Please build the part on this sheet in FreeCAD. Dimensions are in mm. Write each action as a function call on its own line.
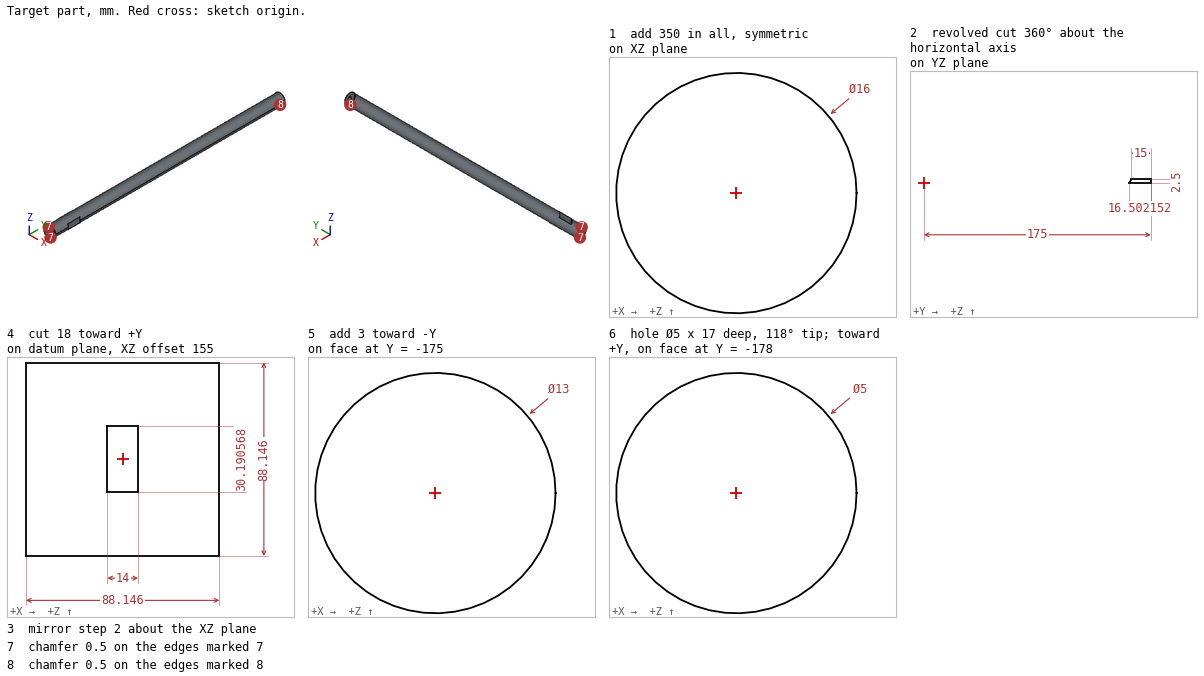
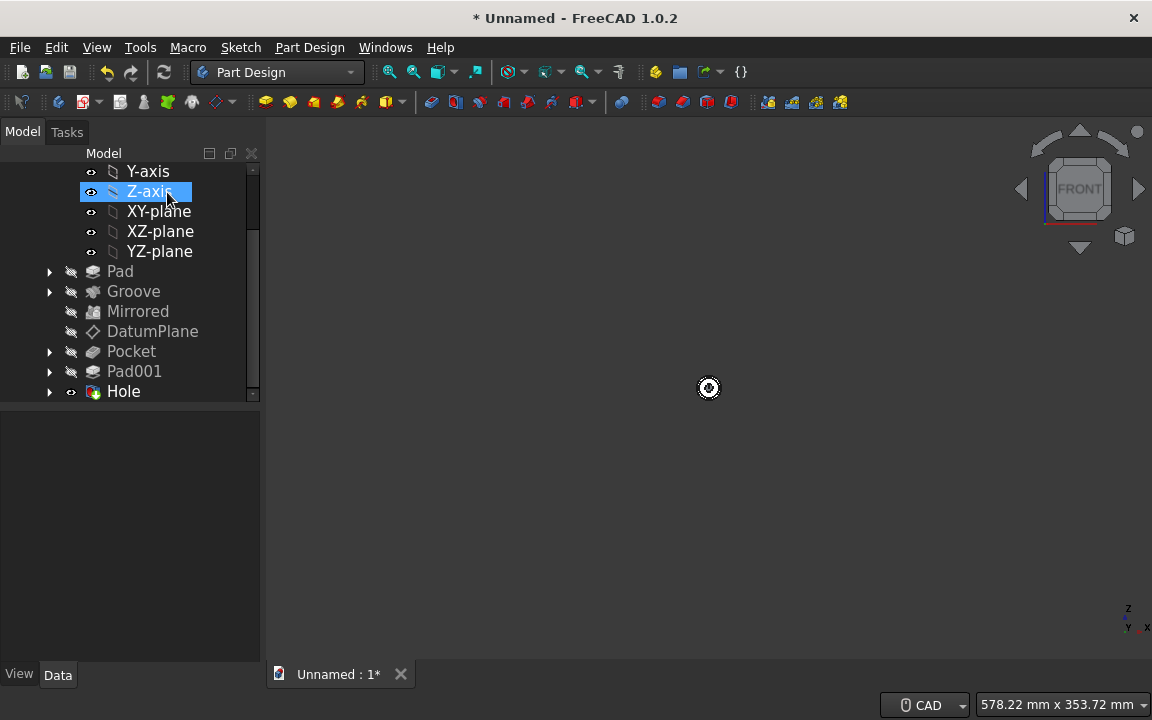
click(390, 72)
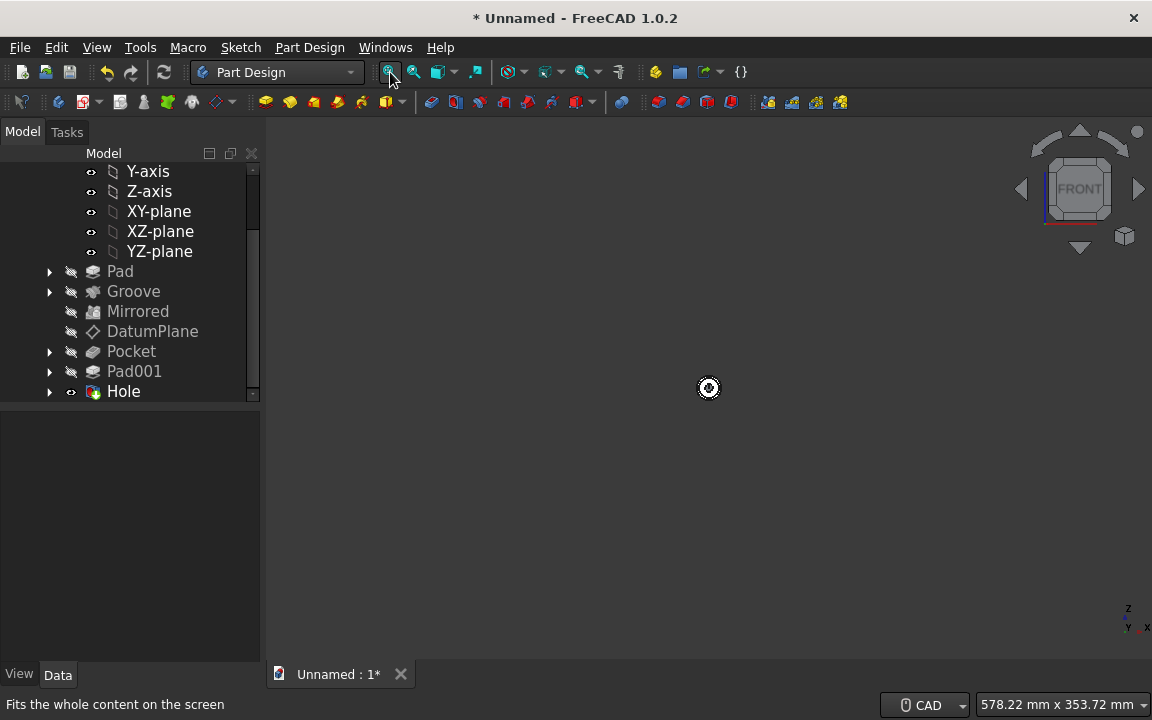
click(699, 387)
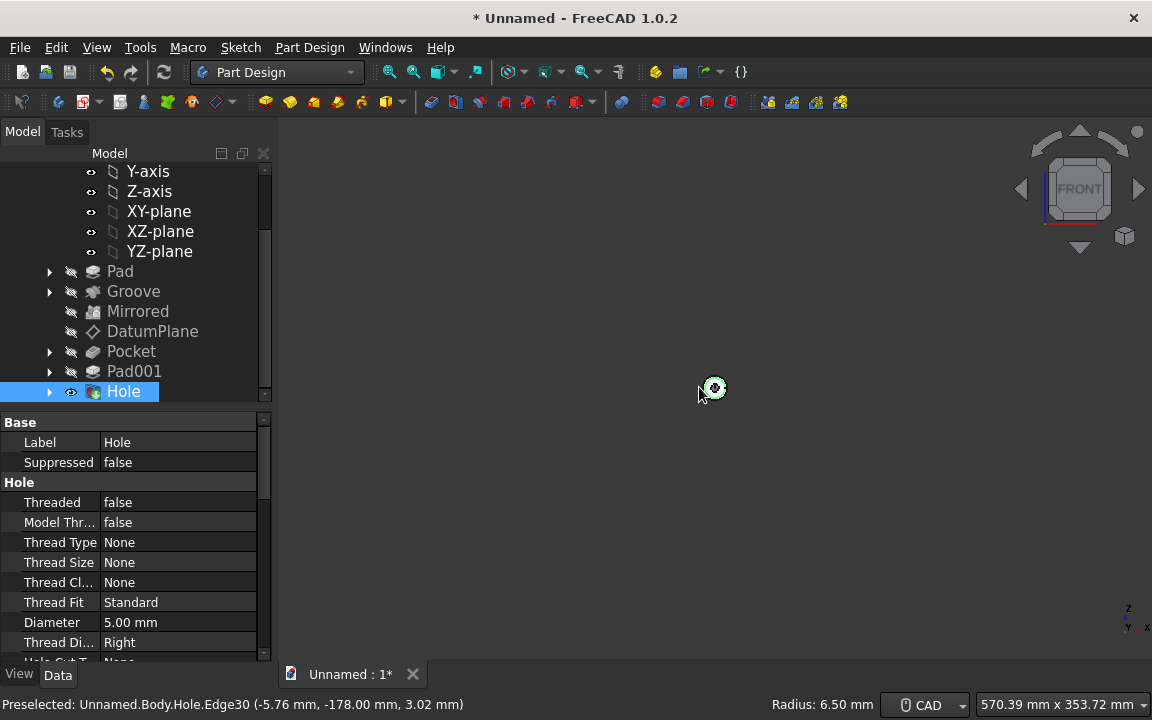
key(0)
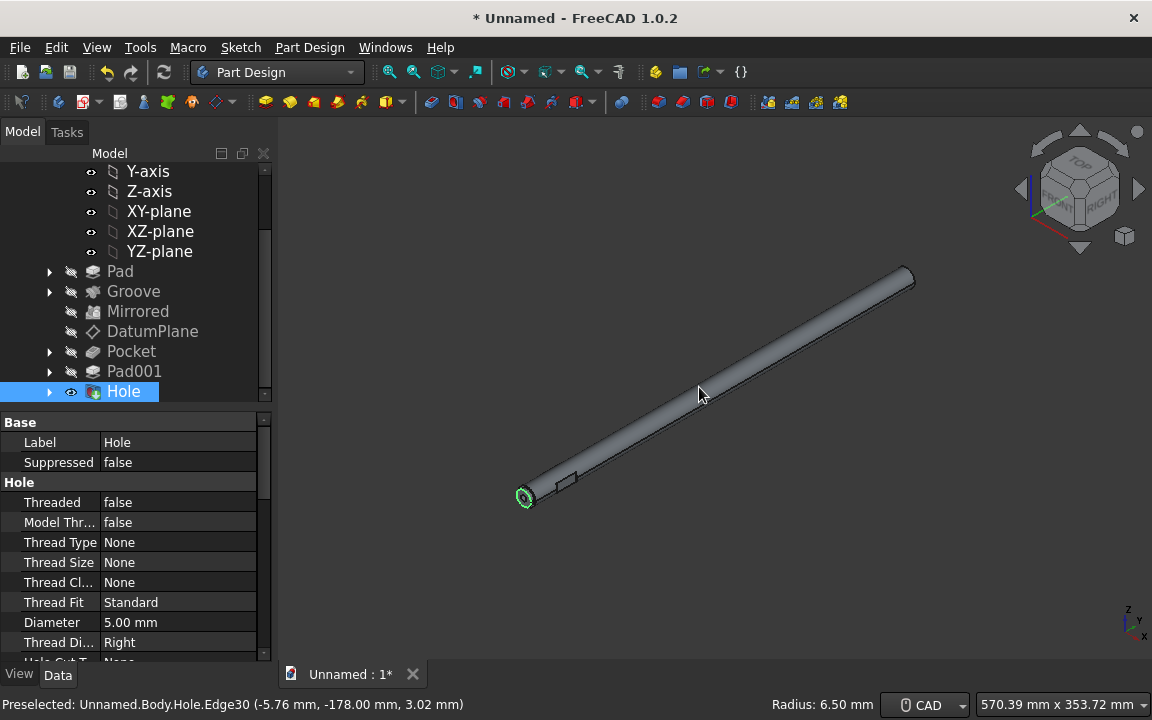
key(2)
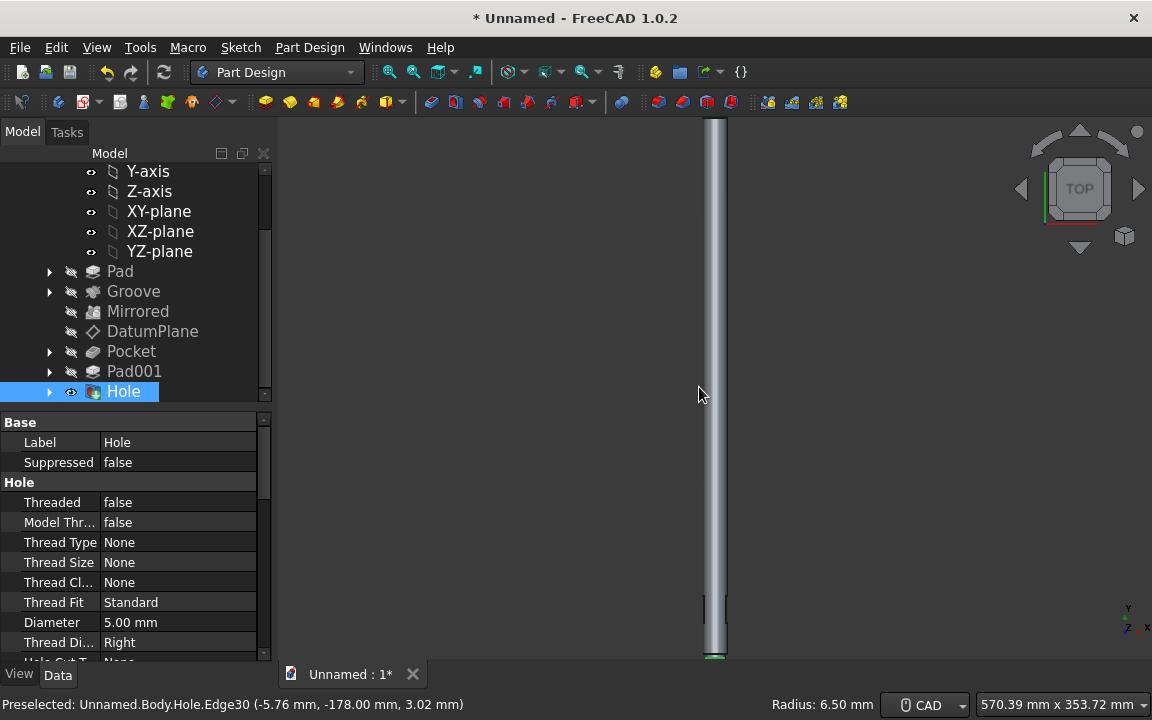
key(1)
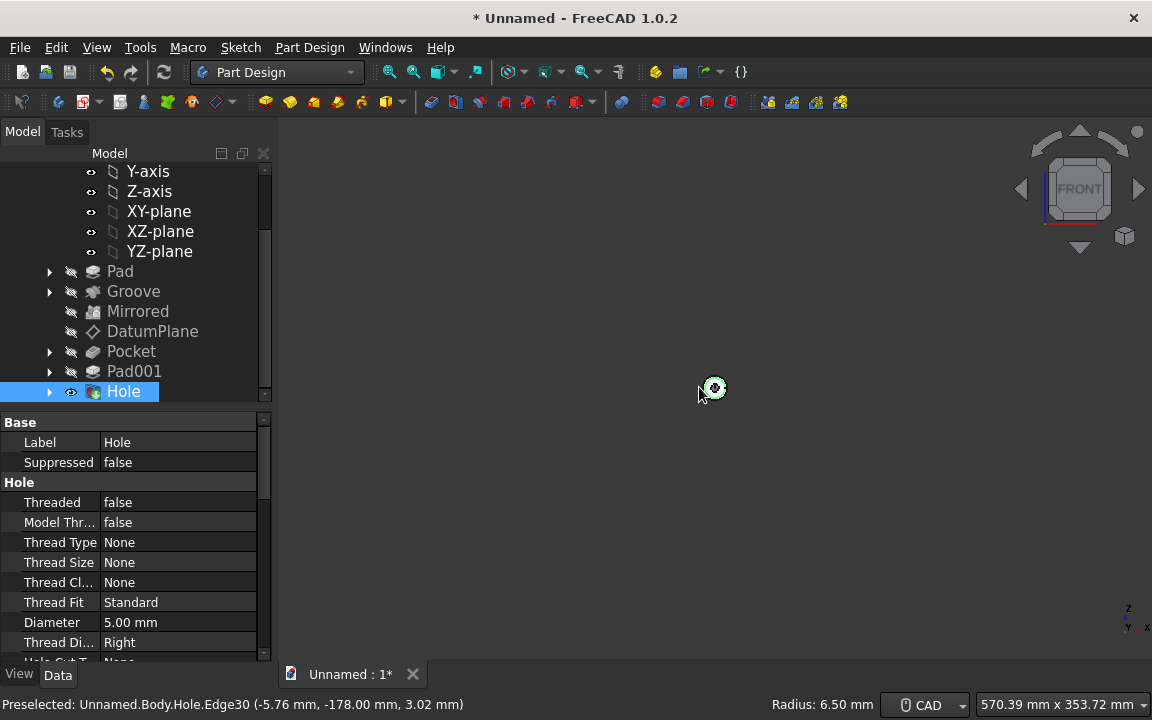
click(390, 72)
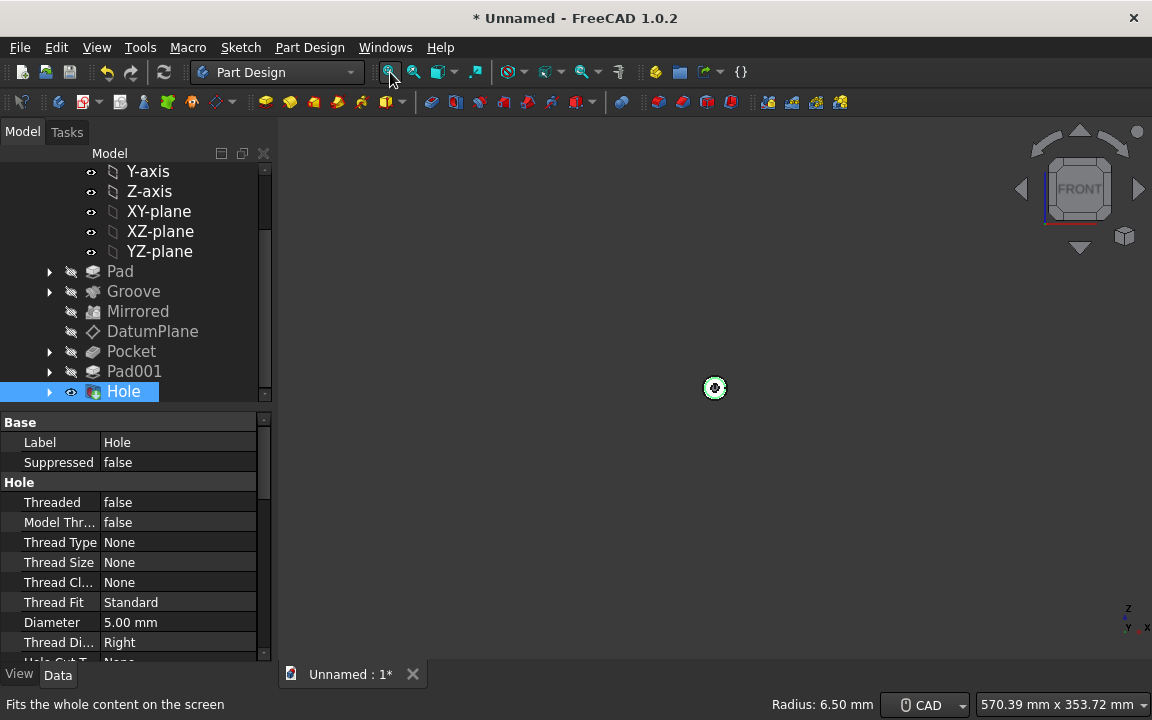
key(3)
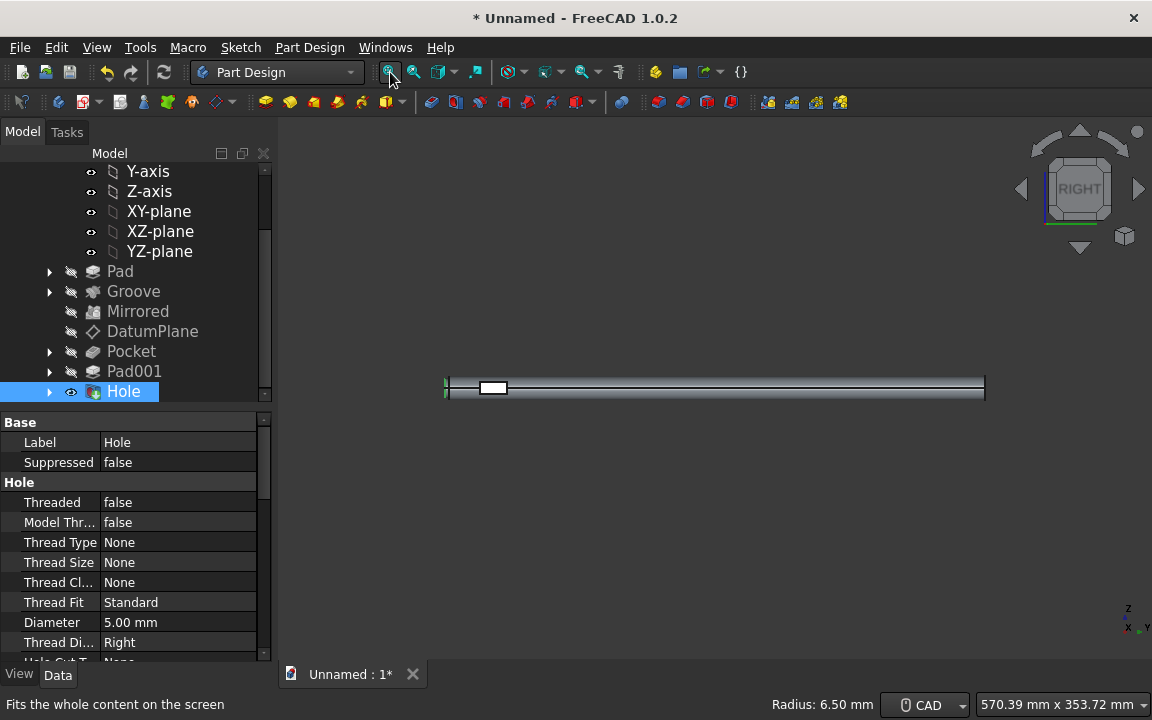
click(449, 380, ctrl)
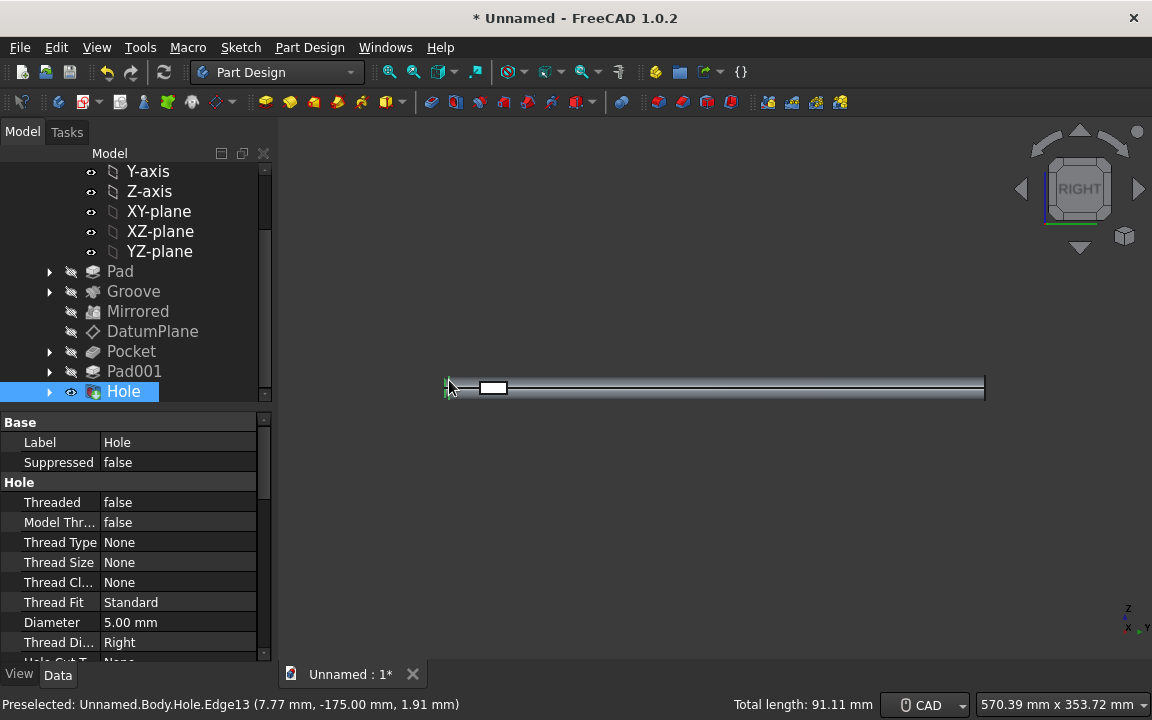
click(684, 102)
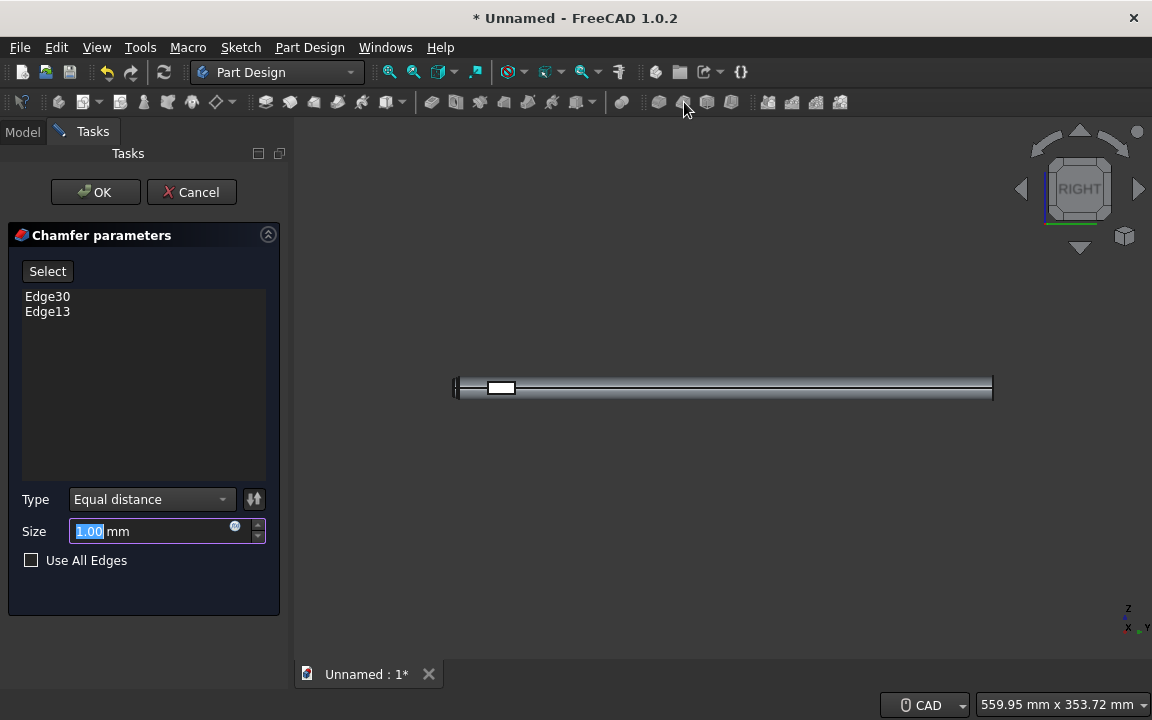
text(0.5)
key(Tab)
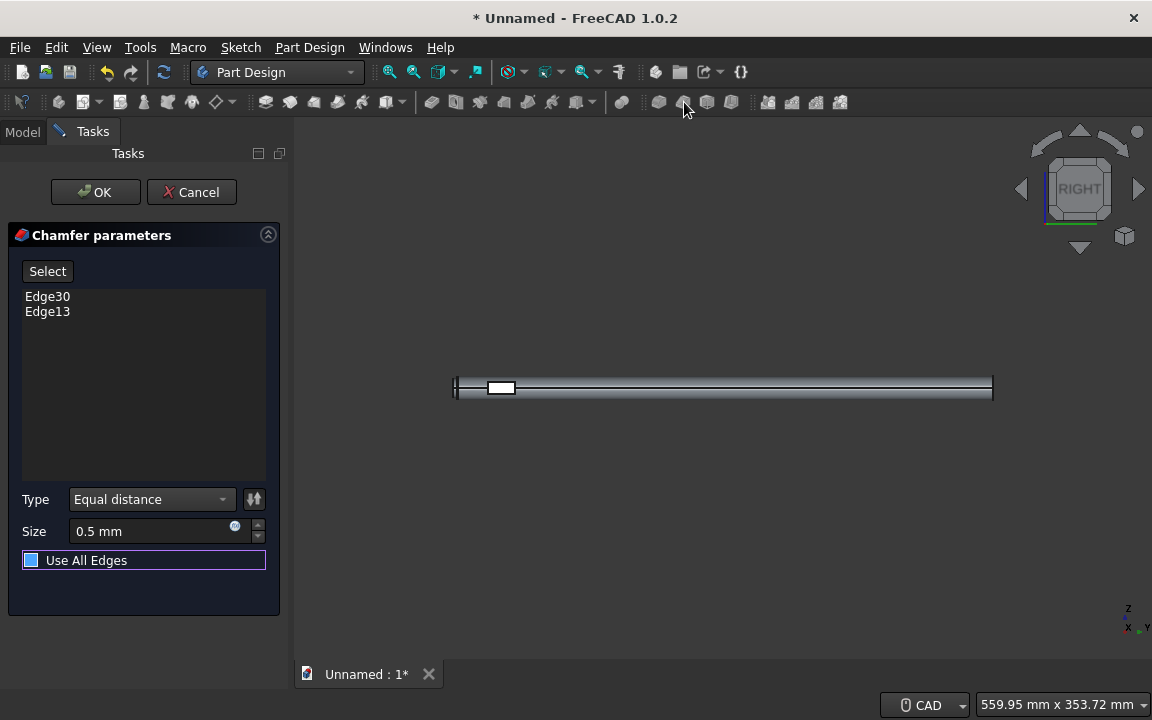
click(96, 192)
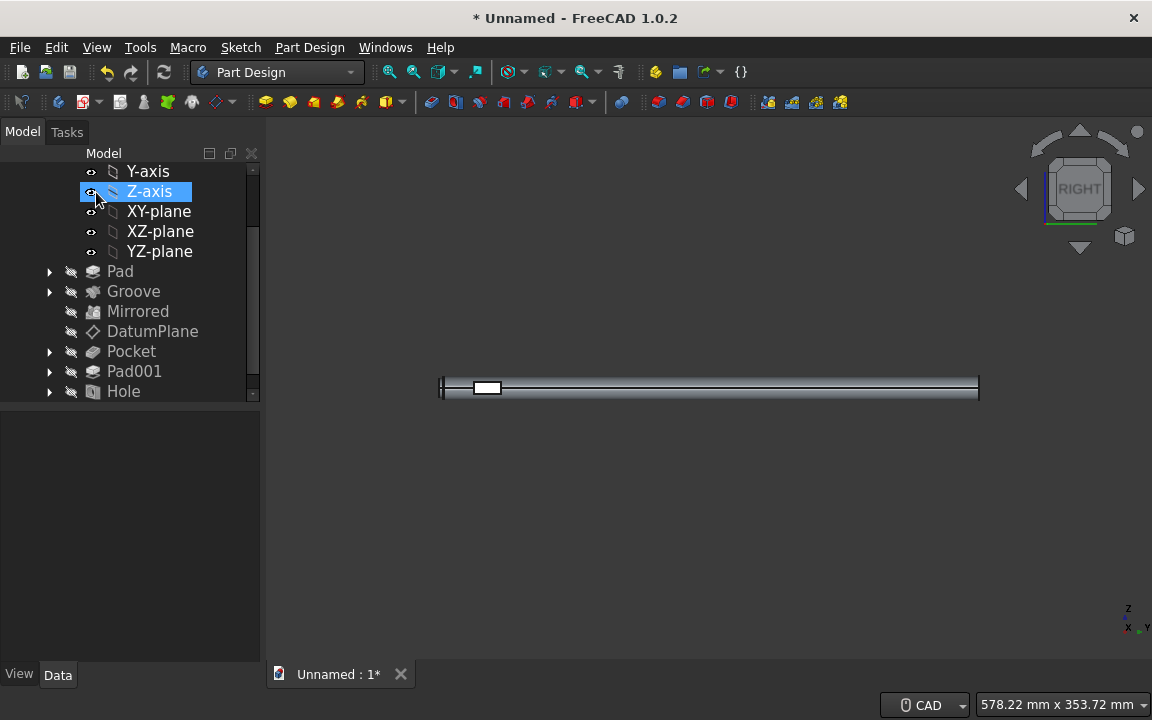
click(979, 380)